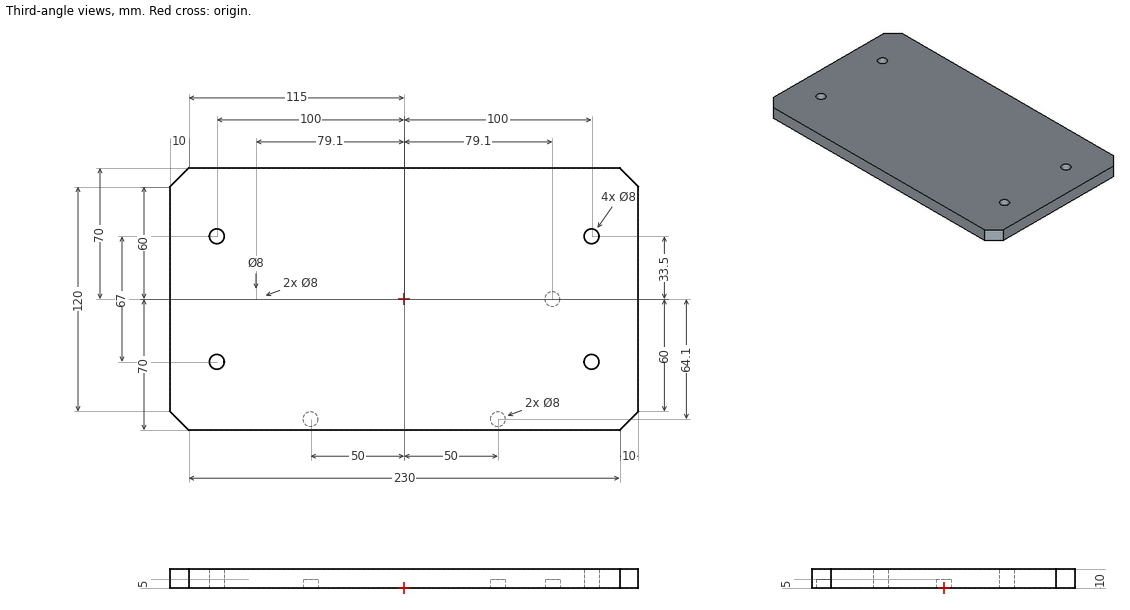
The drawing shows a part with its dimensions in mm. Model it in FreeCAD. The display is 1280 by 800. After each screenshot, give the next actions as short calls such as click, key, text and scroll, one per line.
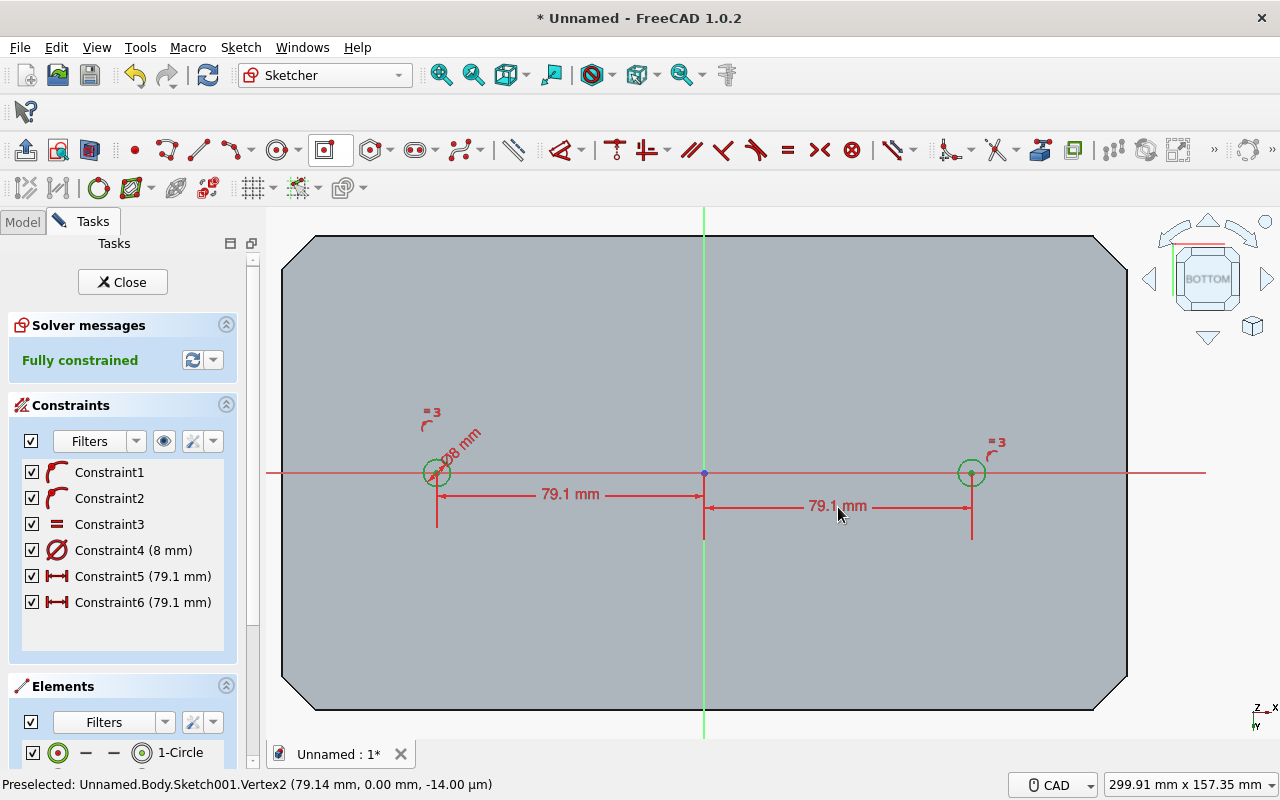
click(123, 282)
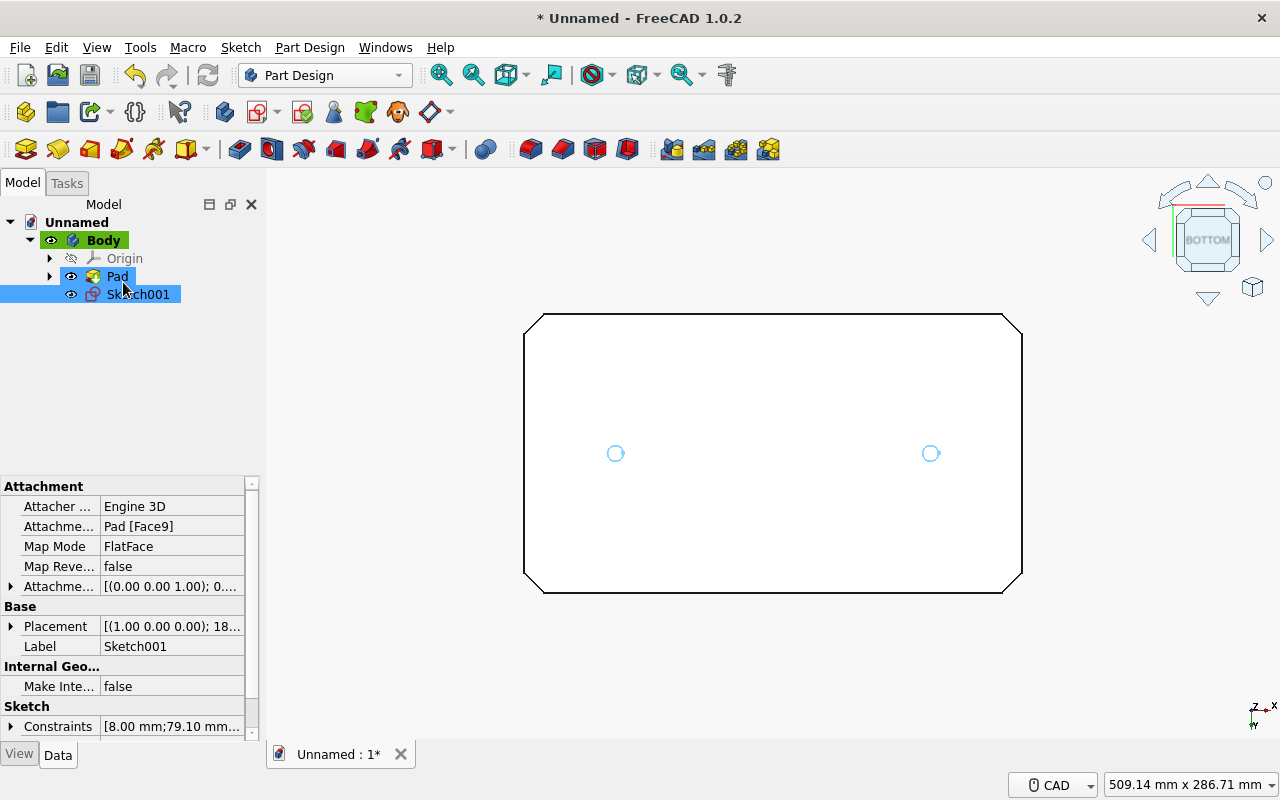
click(240, 150)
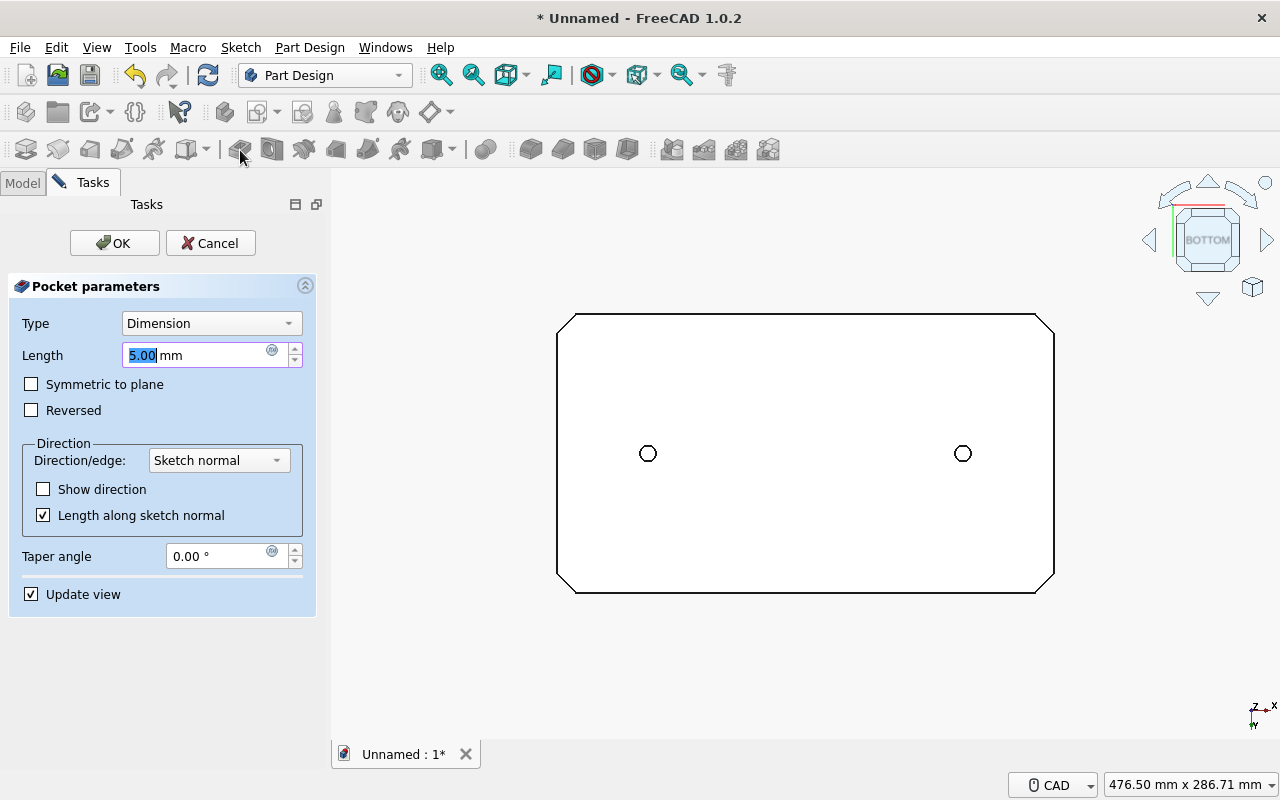
text(5)
key(Tab)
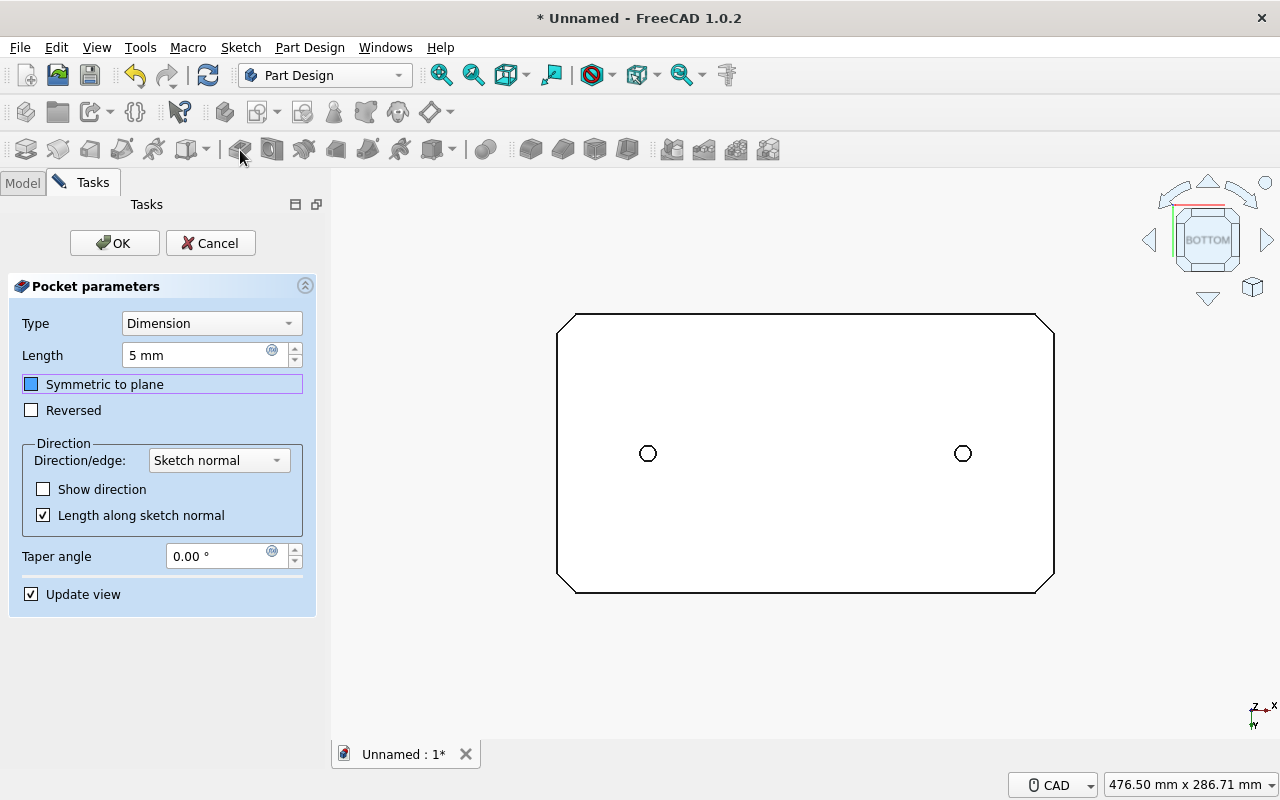
click(115, 243)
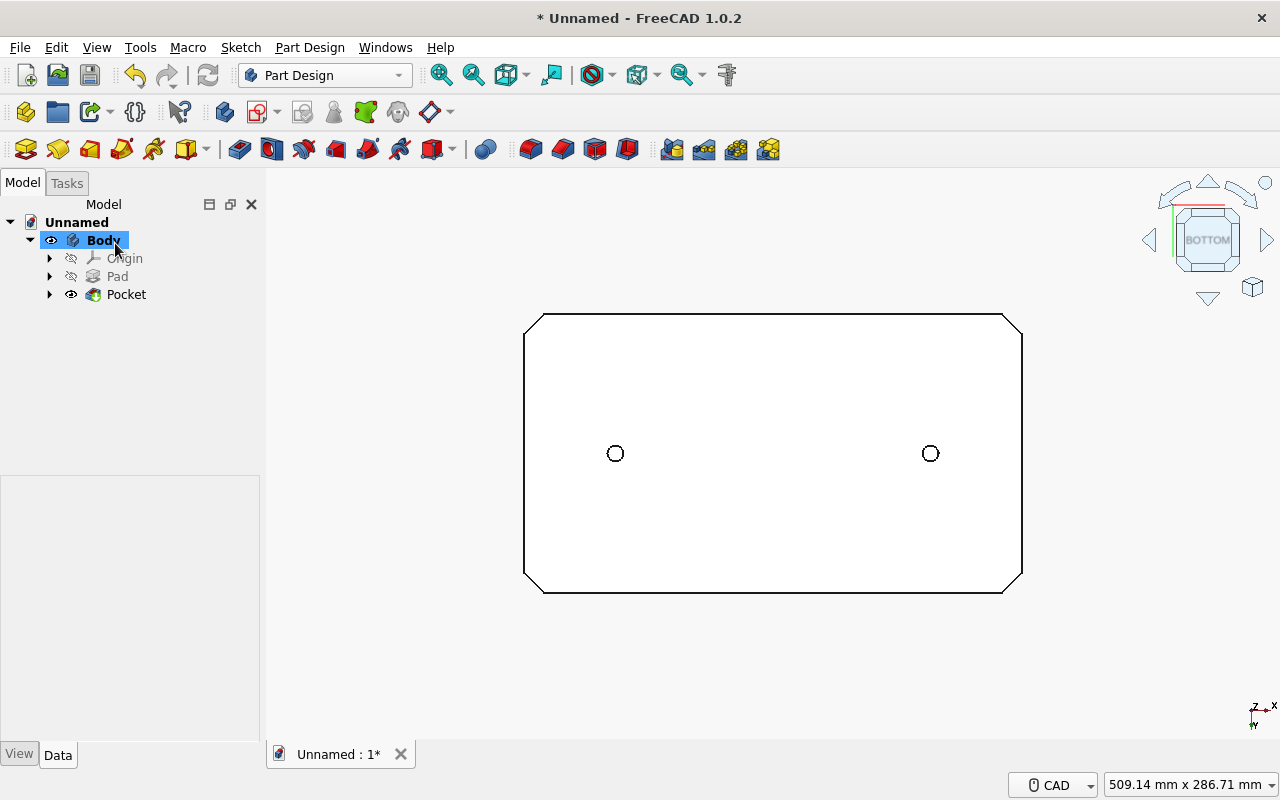
click(773, 453)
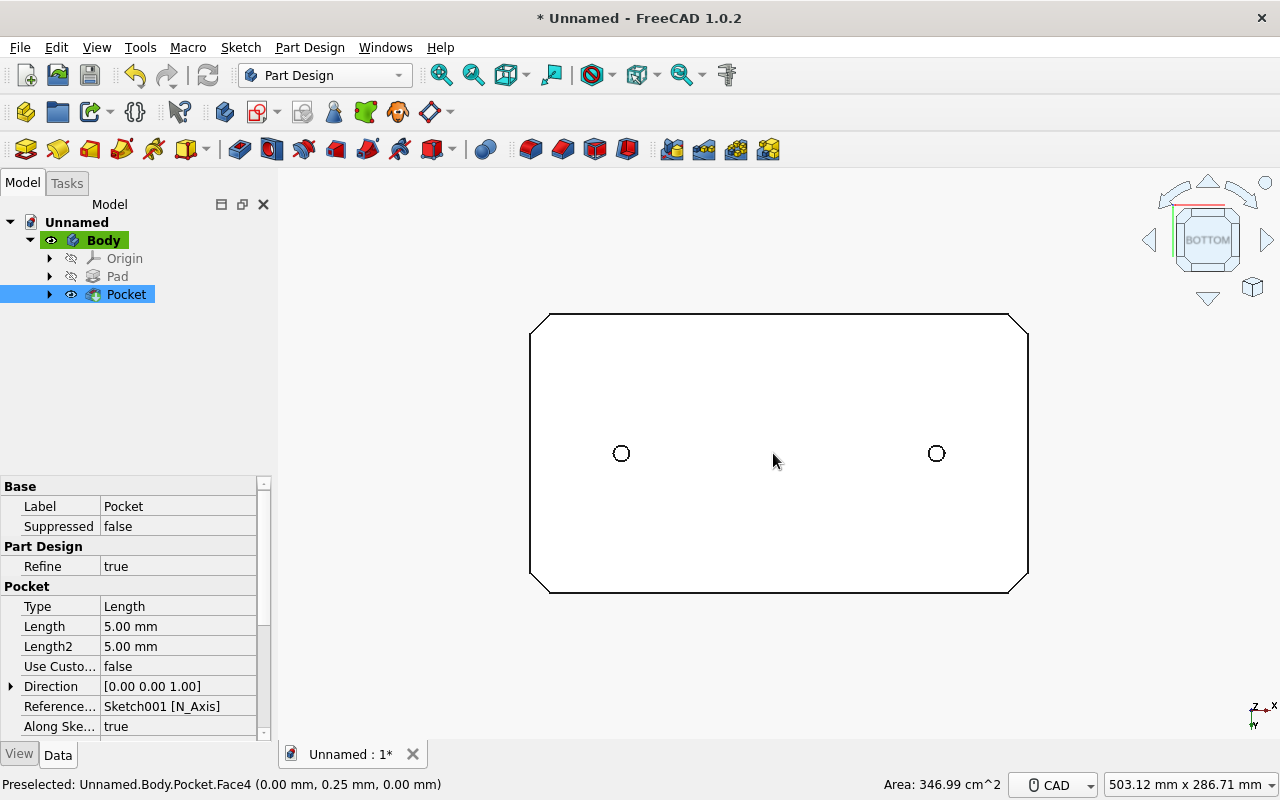
click(258, 112)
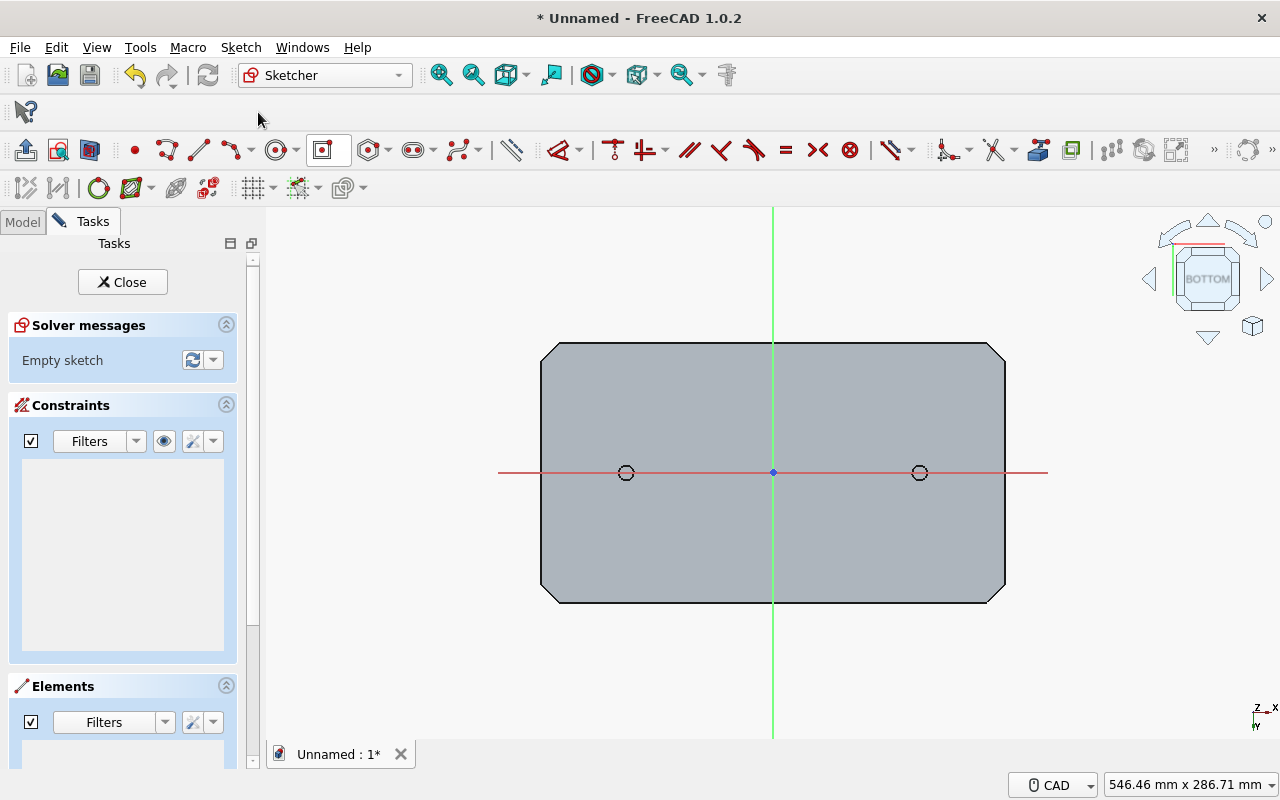
scroll(622, 473, up, 15)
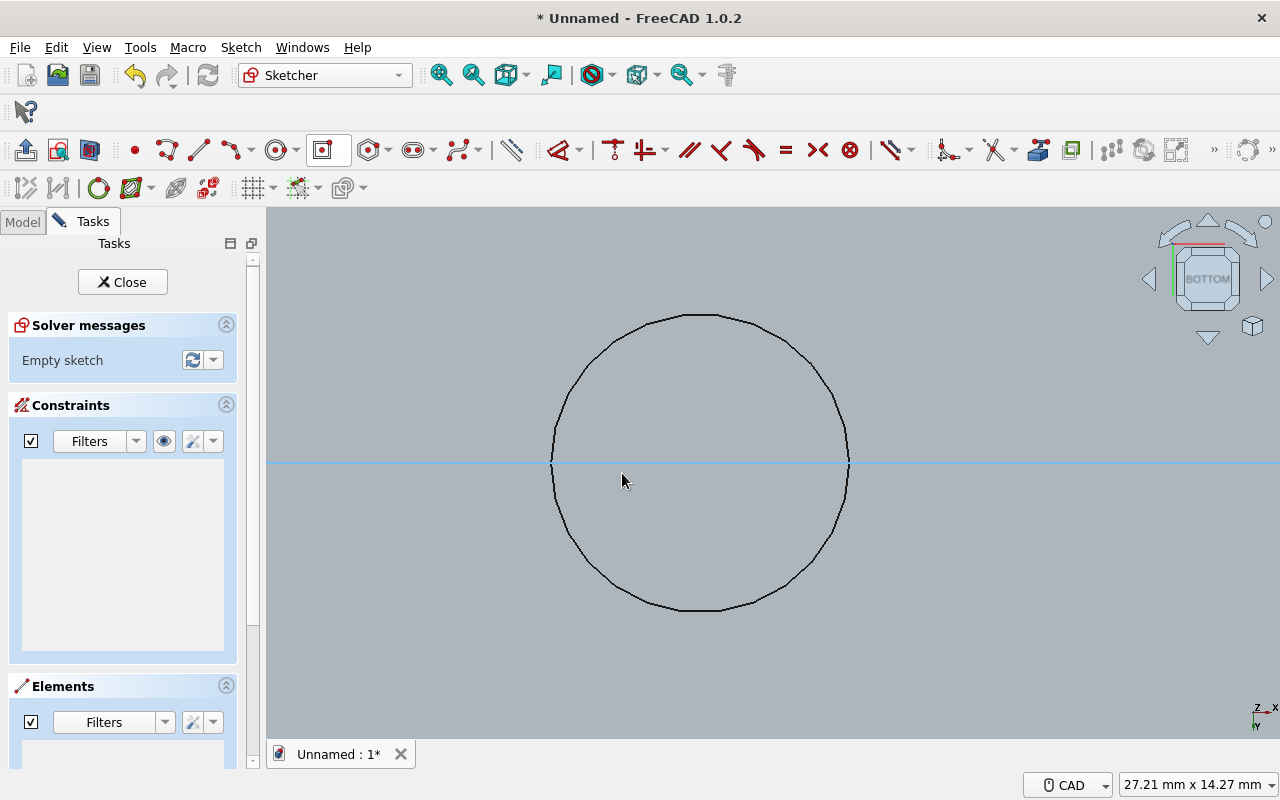
click(276, 150)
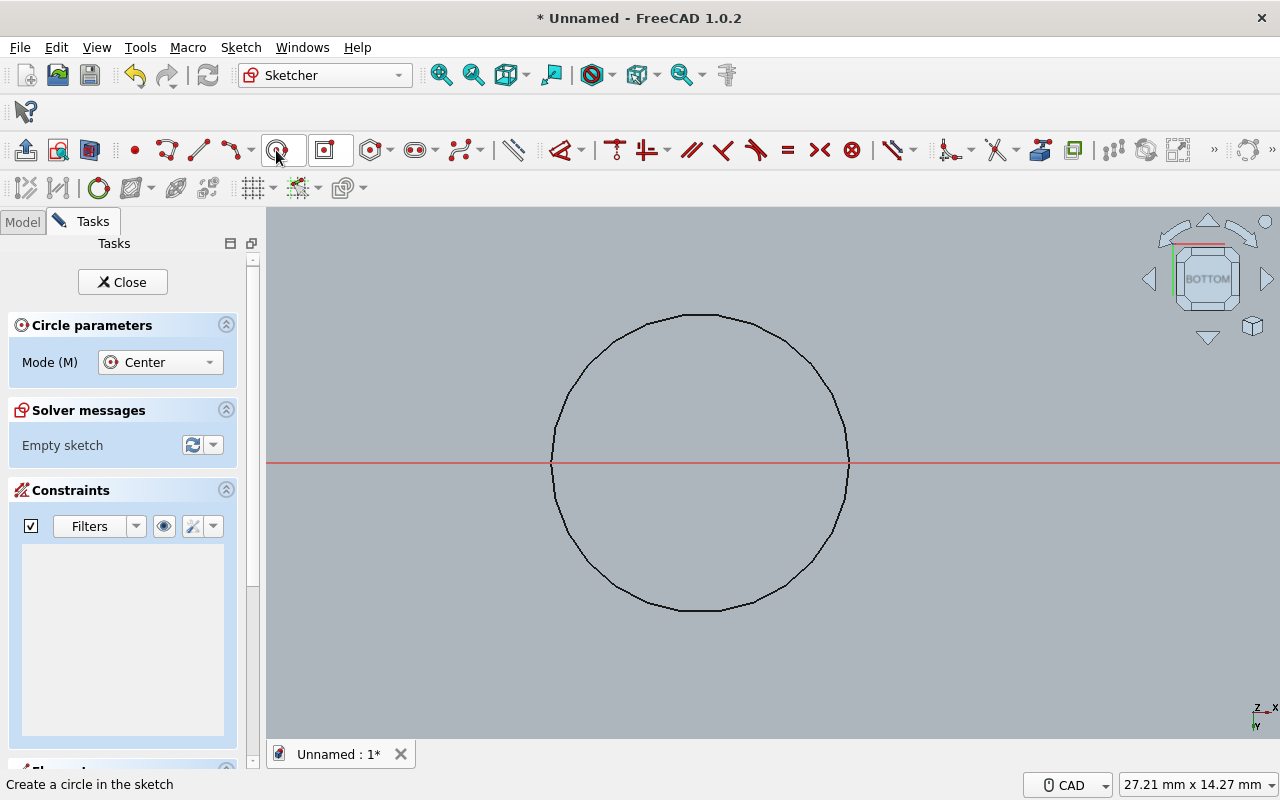
click(700, 463)
click(806, 358)
key(Escape)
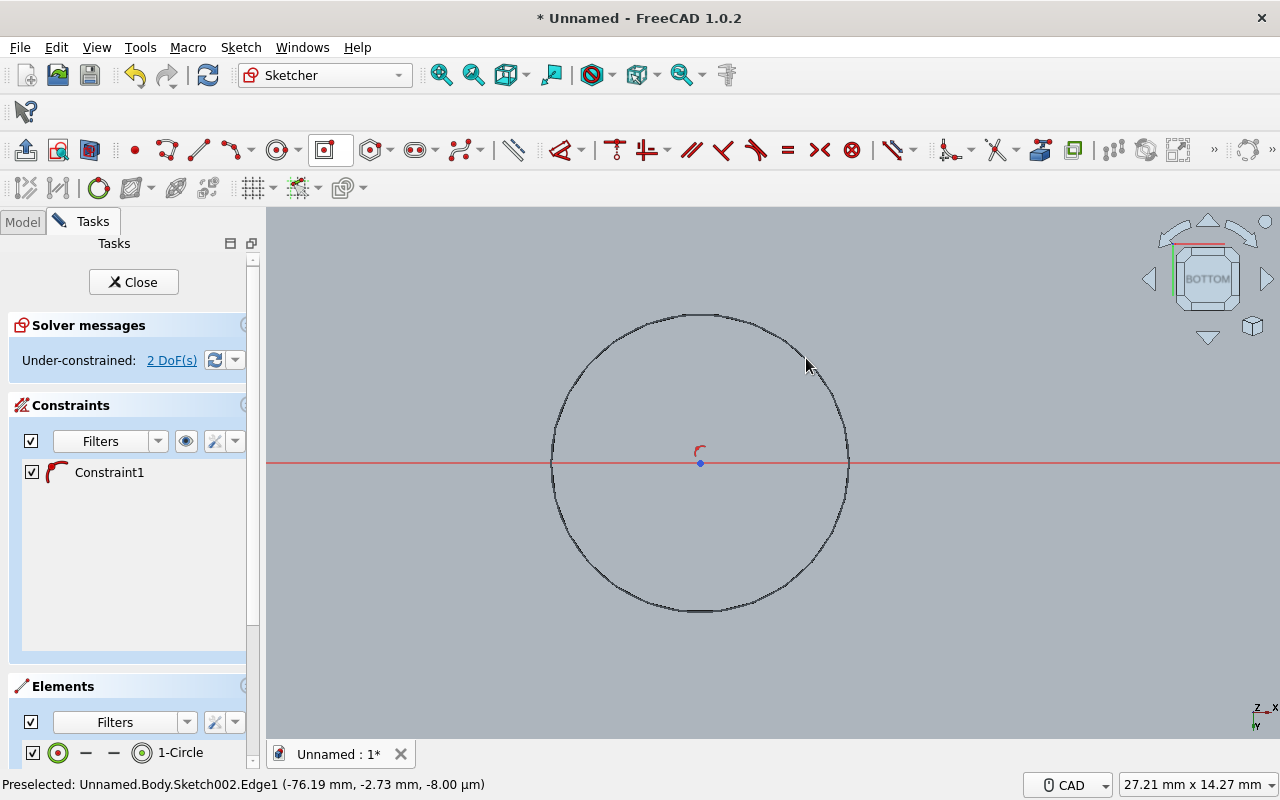
click(560, 150)